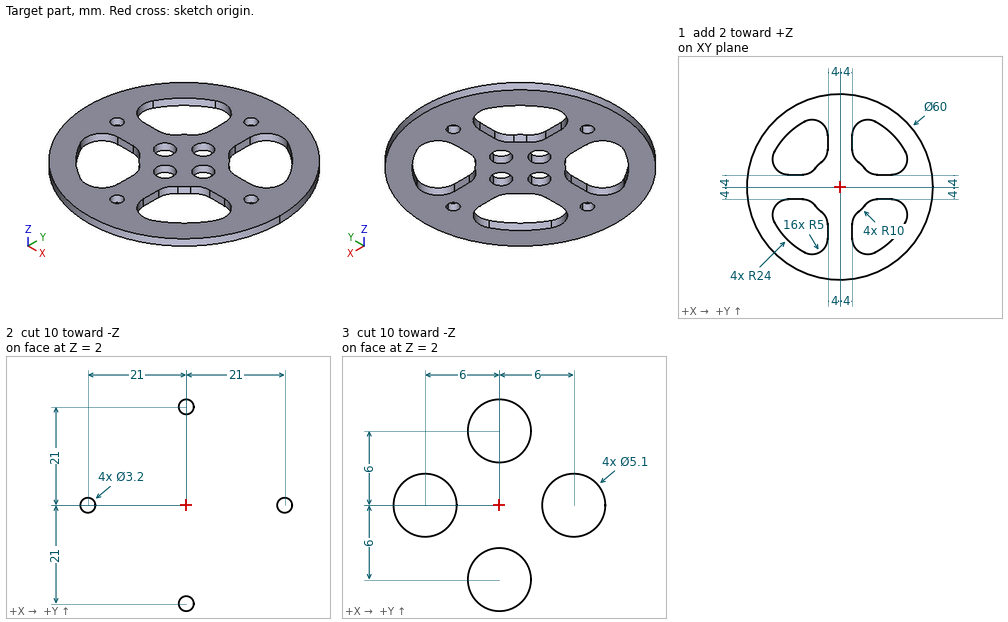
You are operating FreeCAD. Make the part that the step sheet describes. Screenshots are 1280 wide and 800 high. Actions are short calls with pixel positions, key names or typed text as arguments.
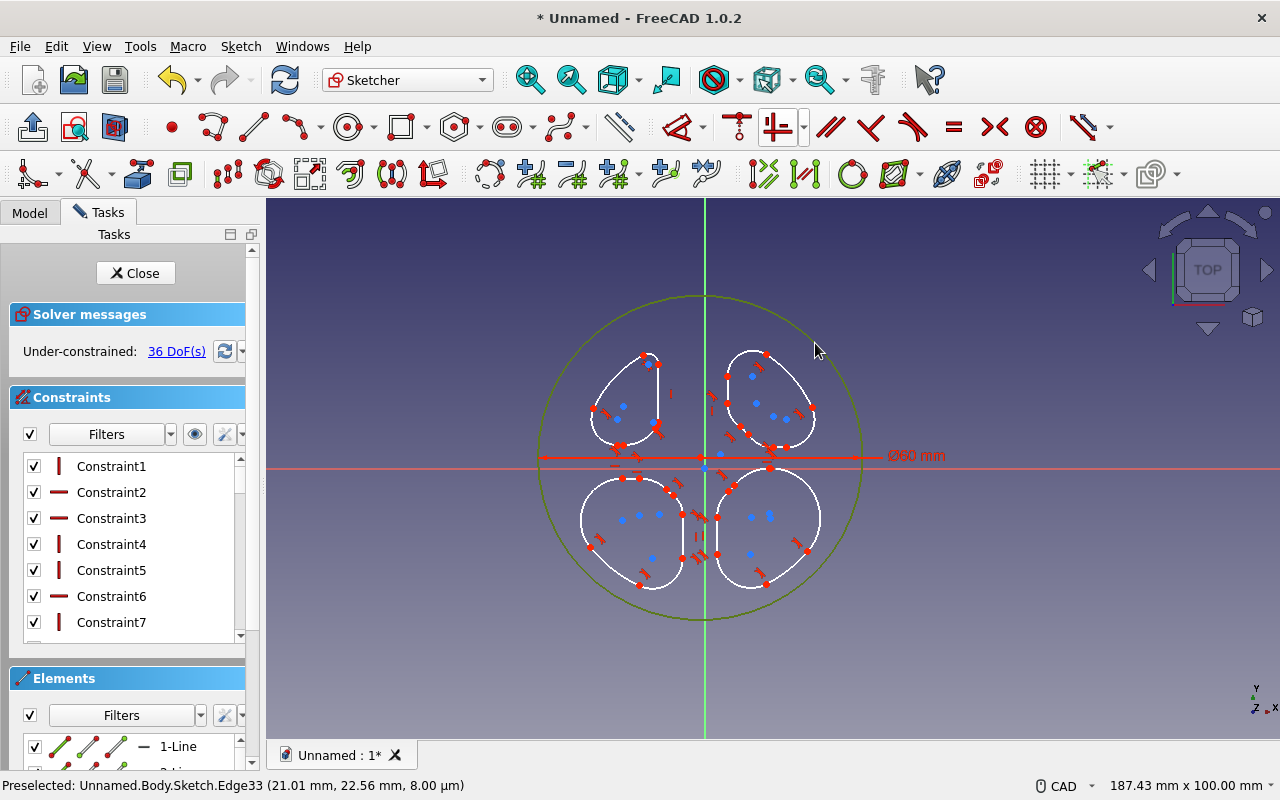
scroll(745, 430, up, 5)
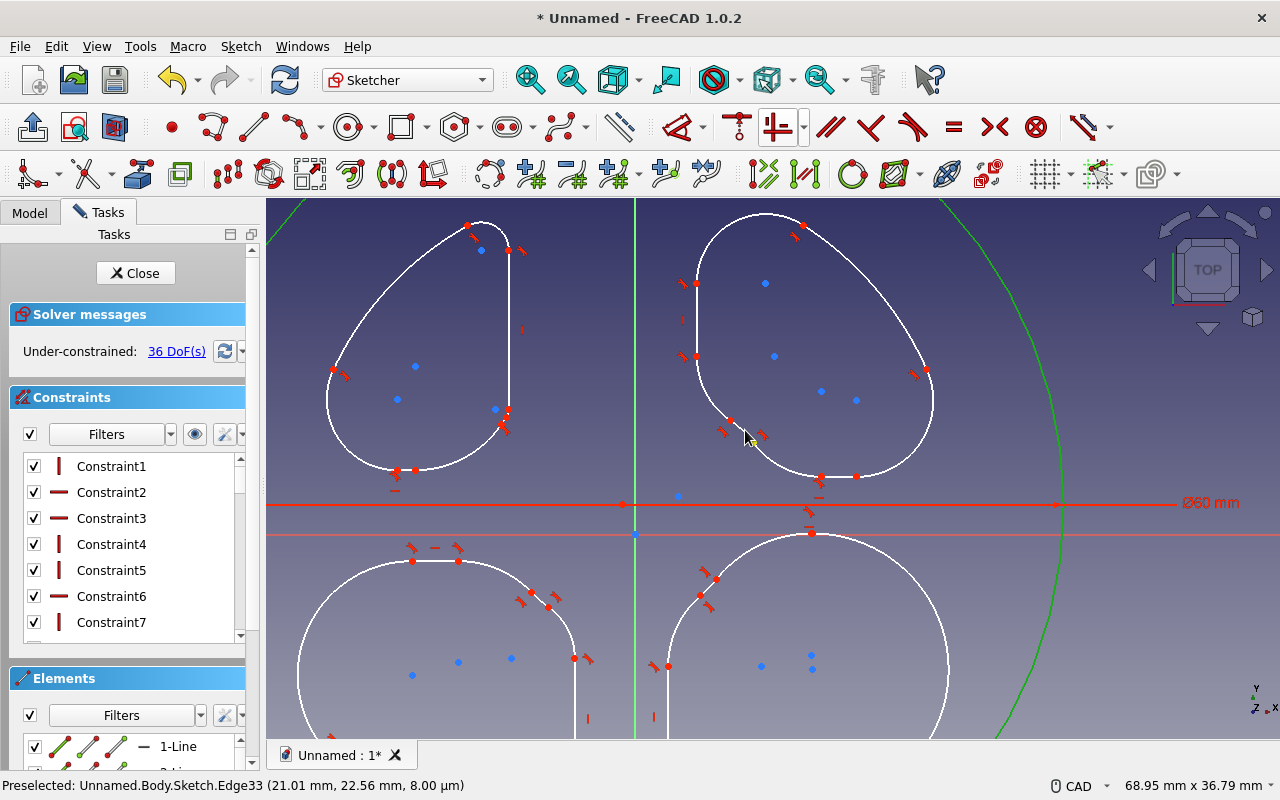
click(743, 431)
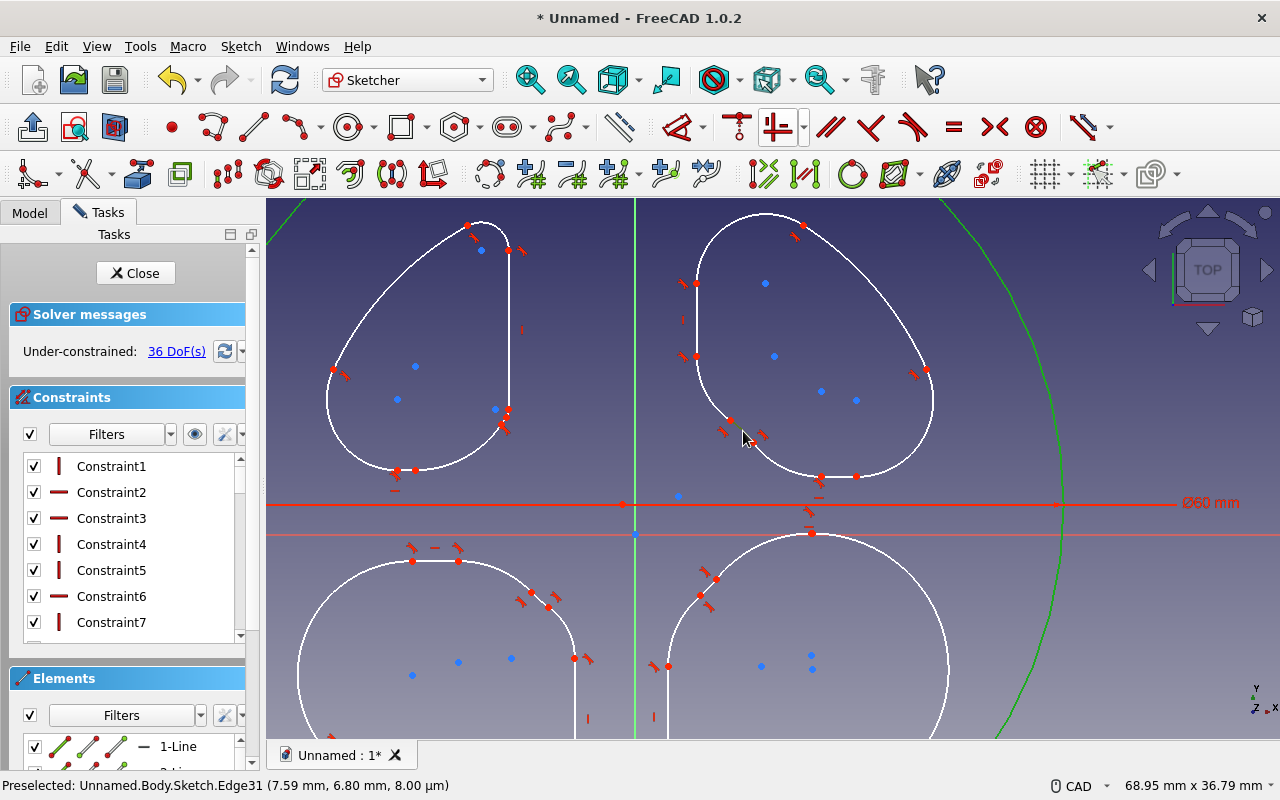
click(737, 128)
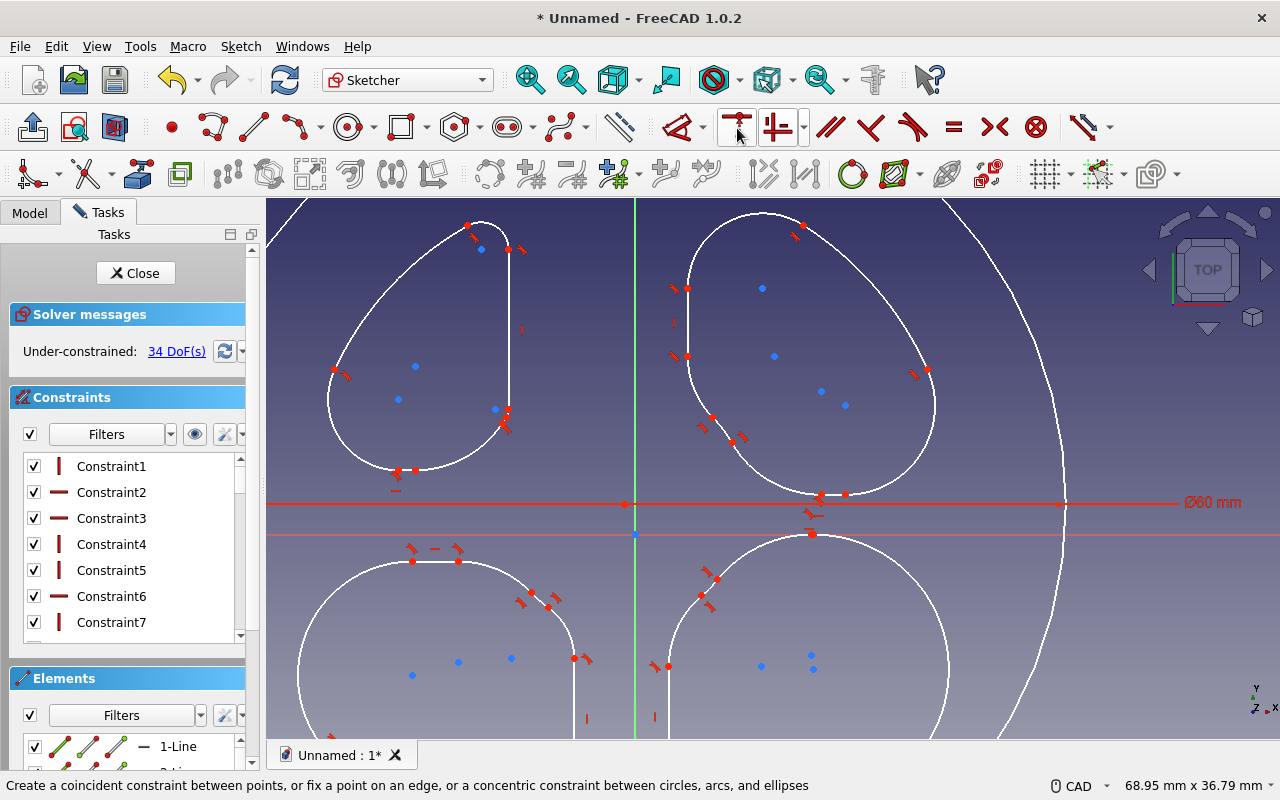
scroll(630, 520, up, 6)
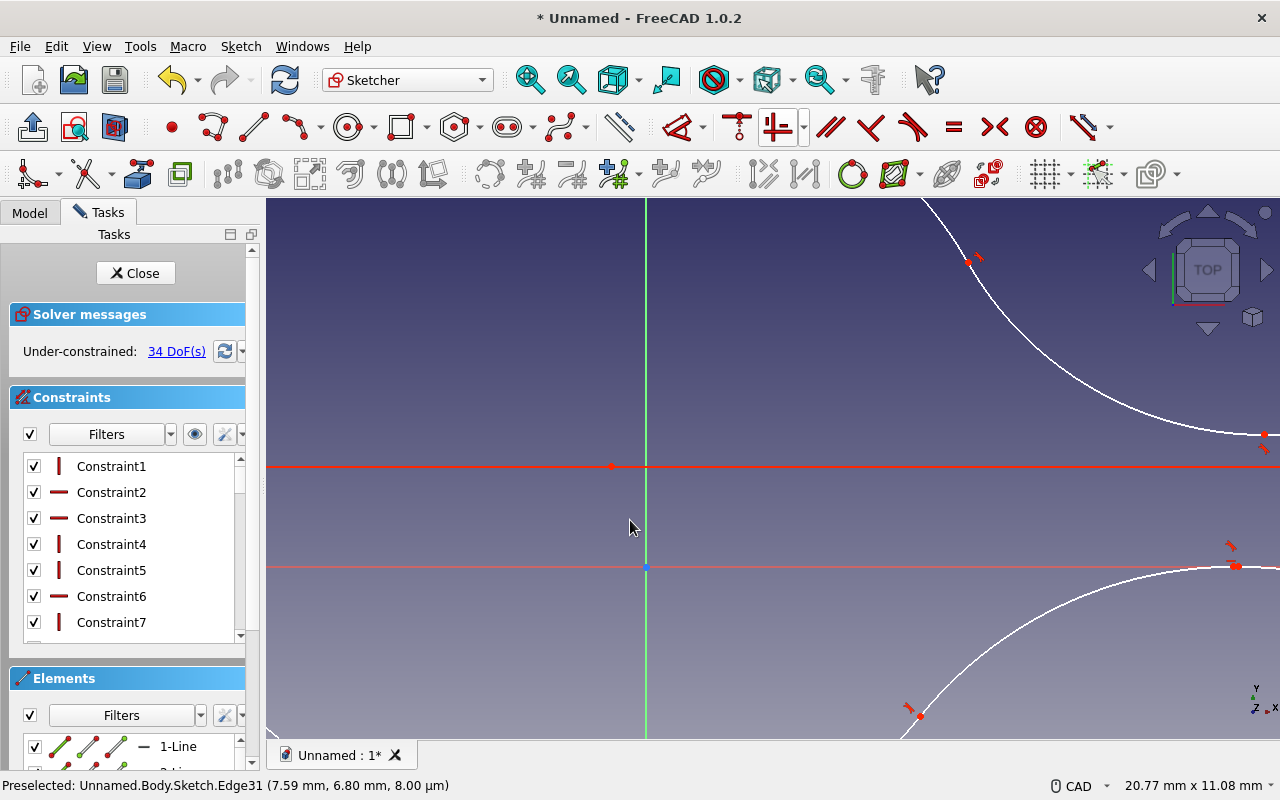
drag(601, 457, 656, 577)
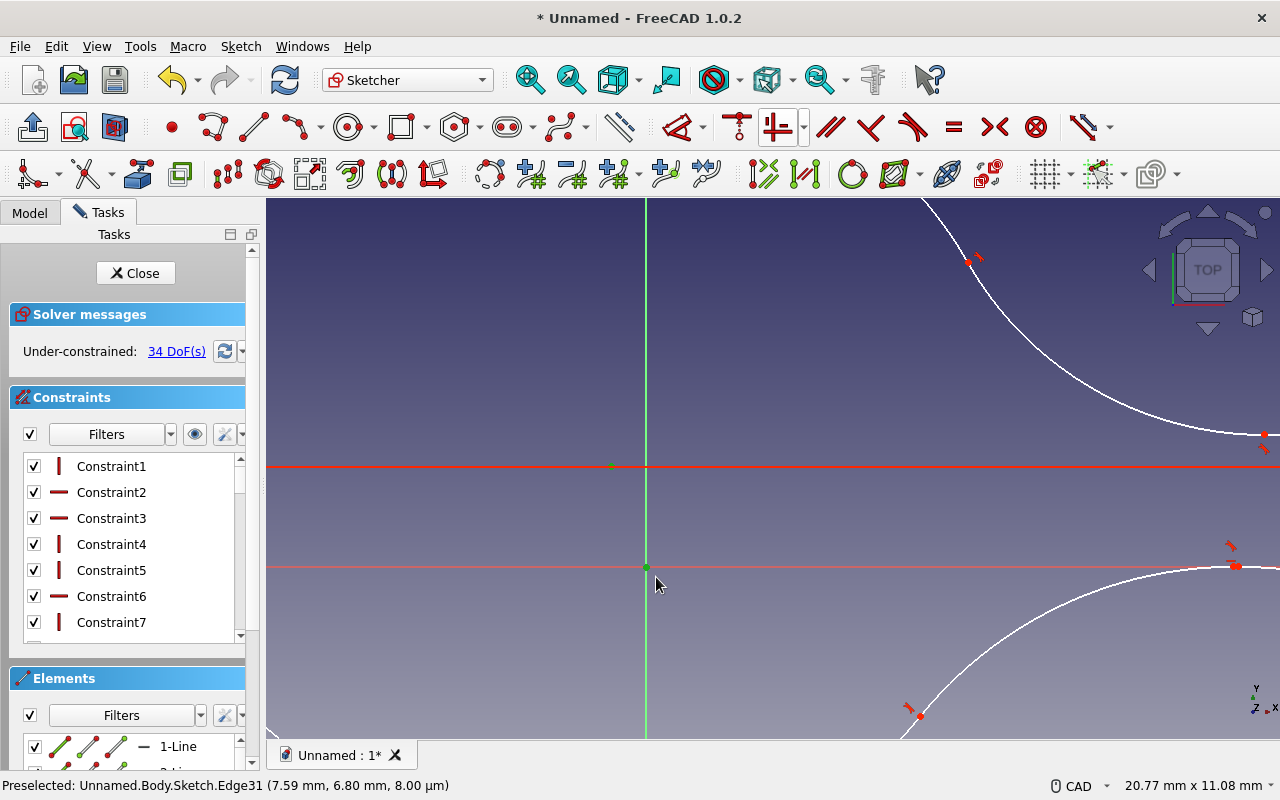
click(737, 128)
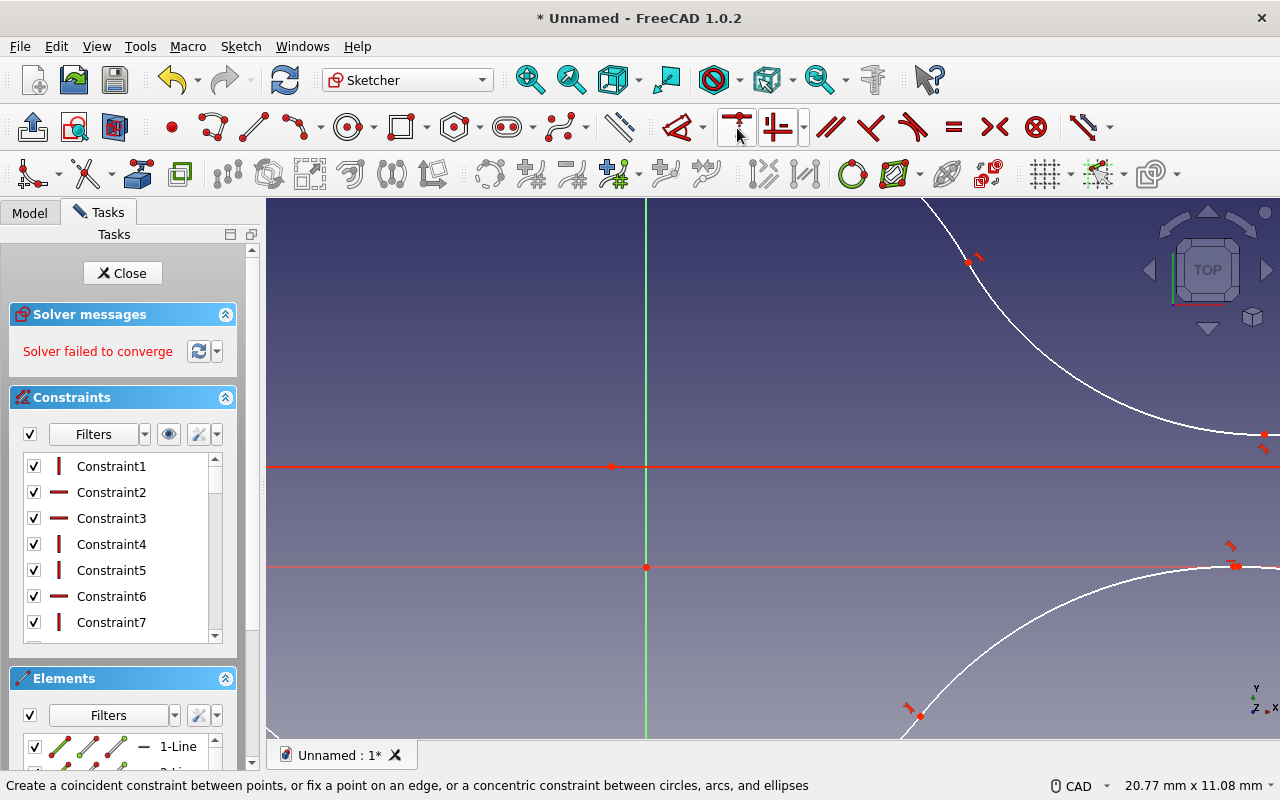
scroll(712, 456, down, 11)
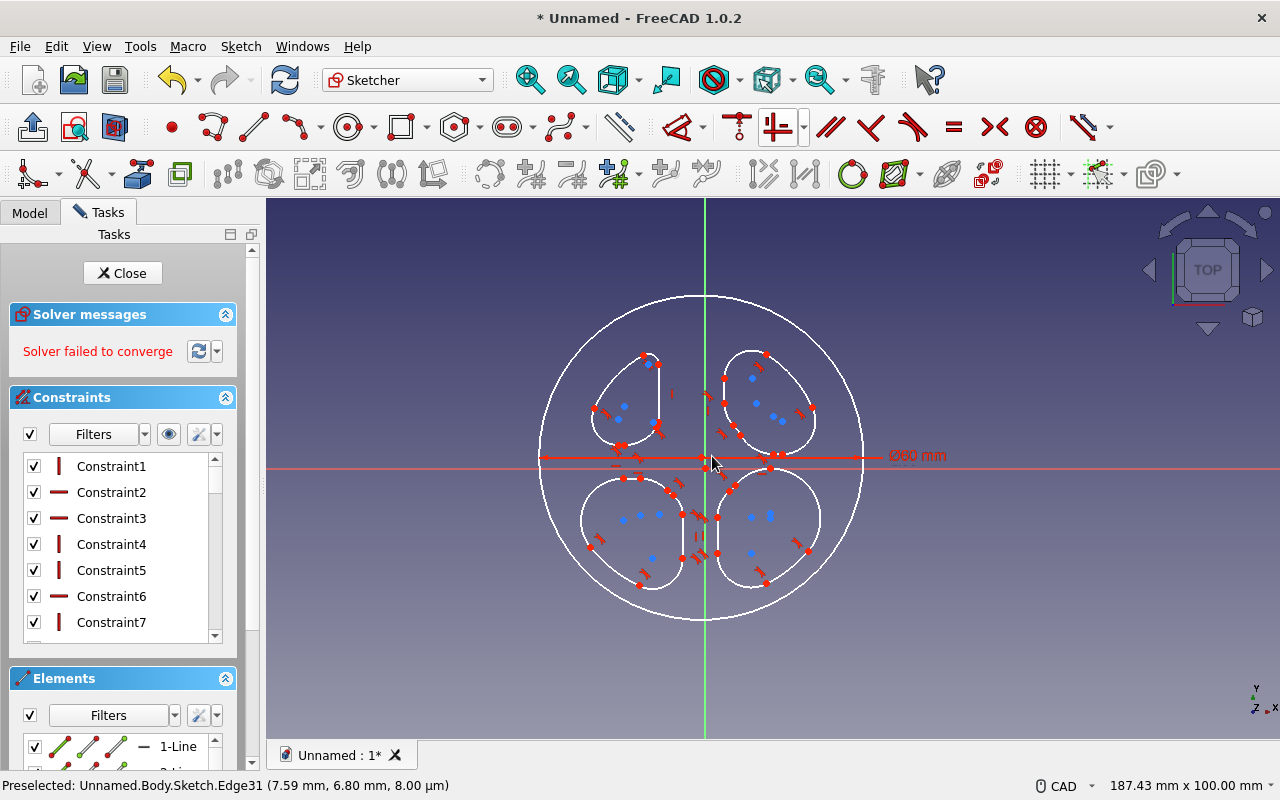
click(657, 589)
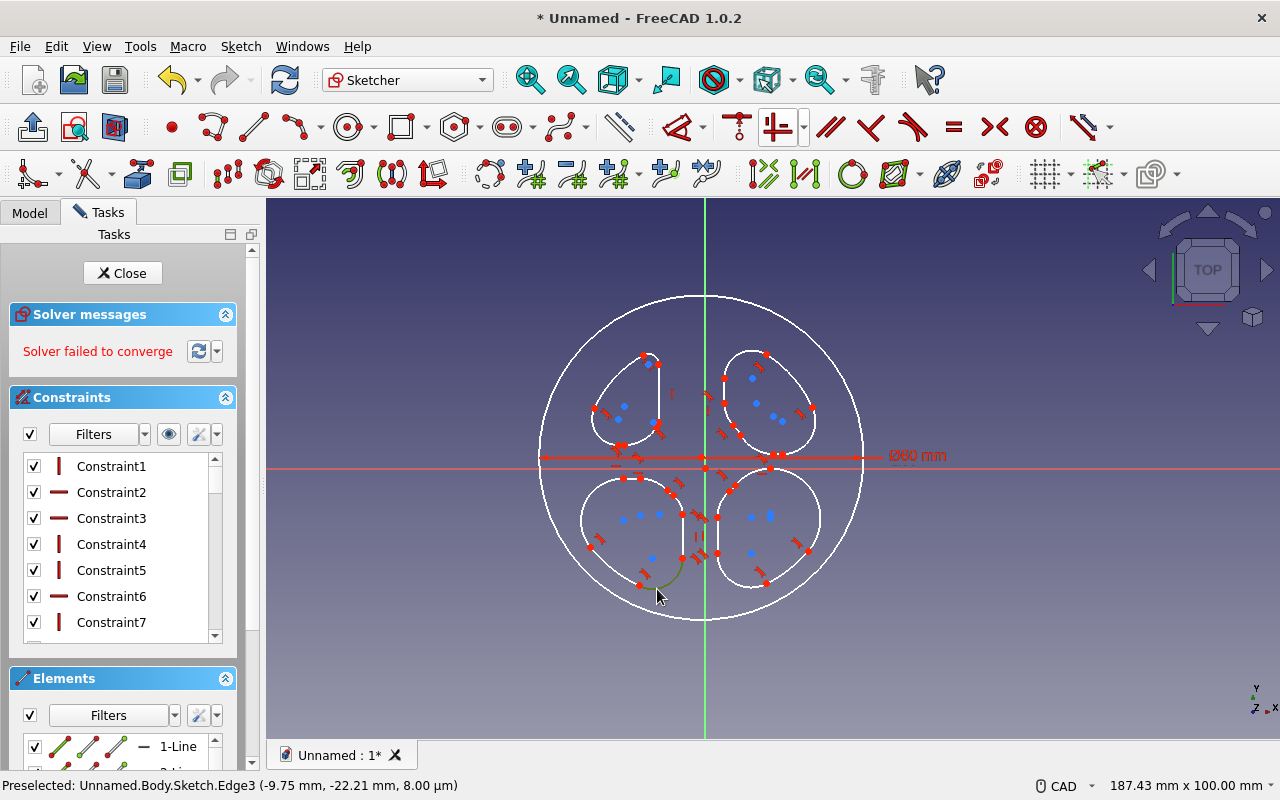
click(597, 488)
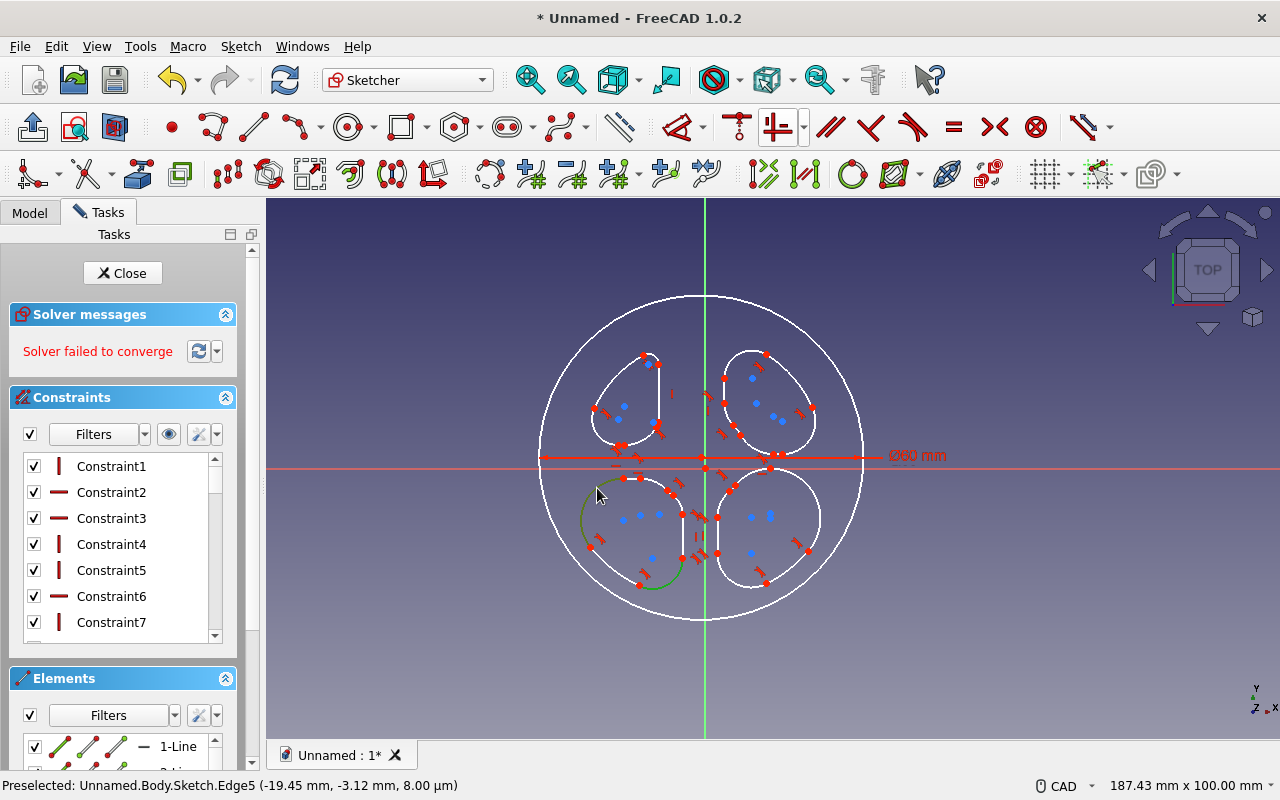
scroll(660, 484, up, 3)